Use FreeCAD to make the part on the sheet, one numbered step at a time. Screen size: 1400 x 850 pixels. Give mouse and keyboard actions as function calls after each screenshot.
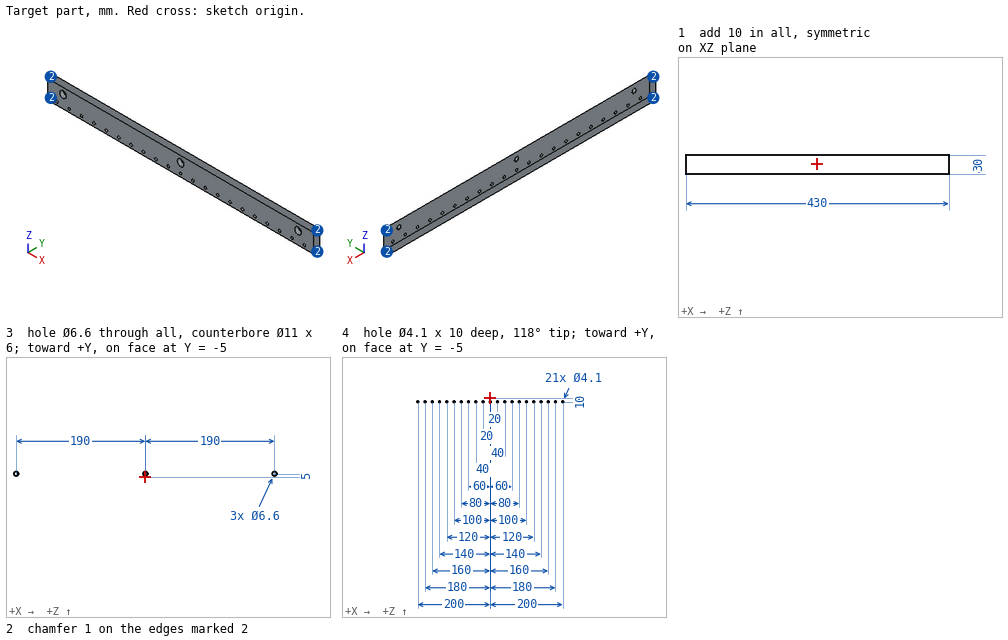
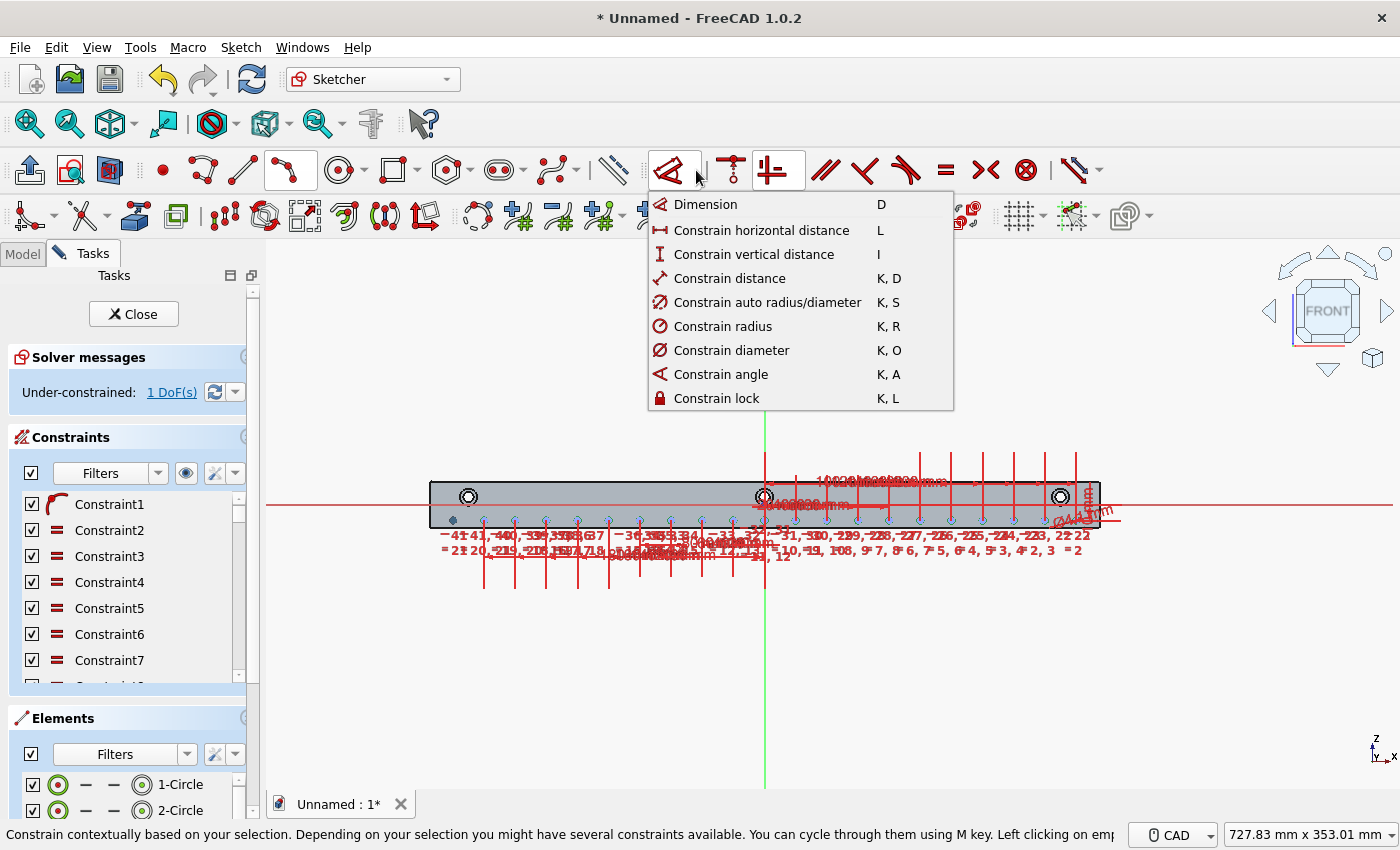
click(801, 230)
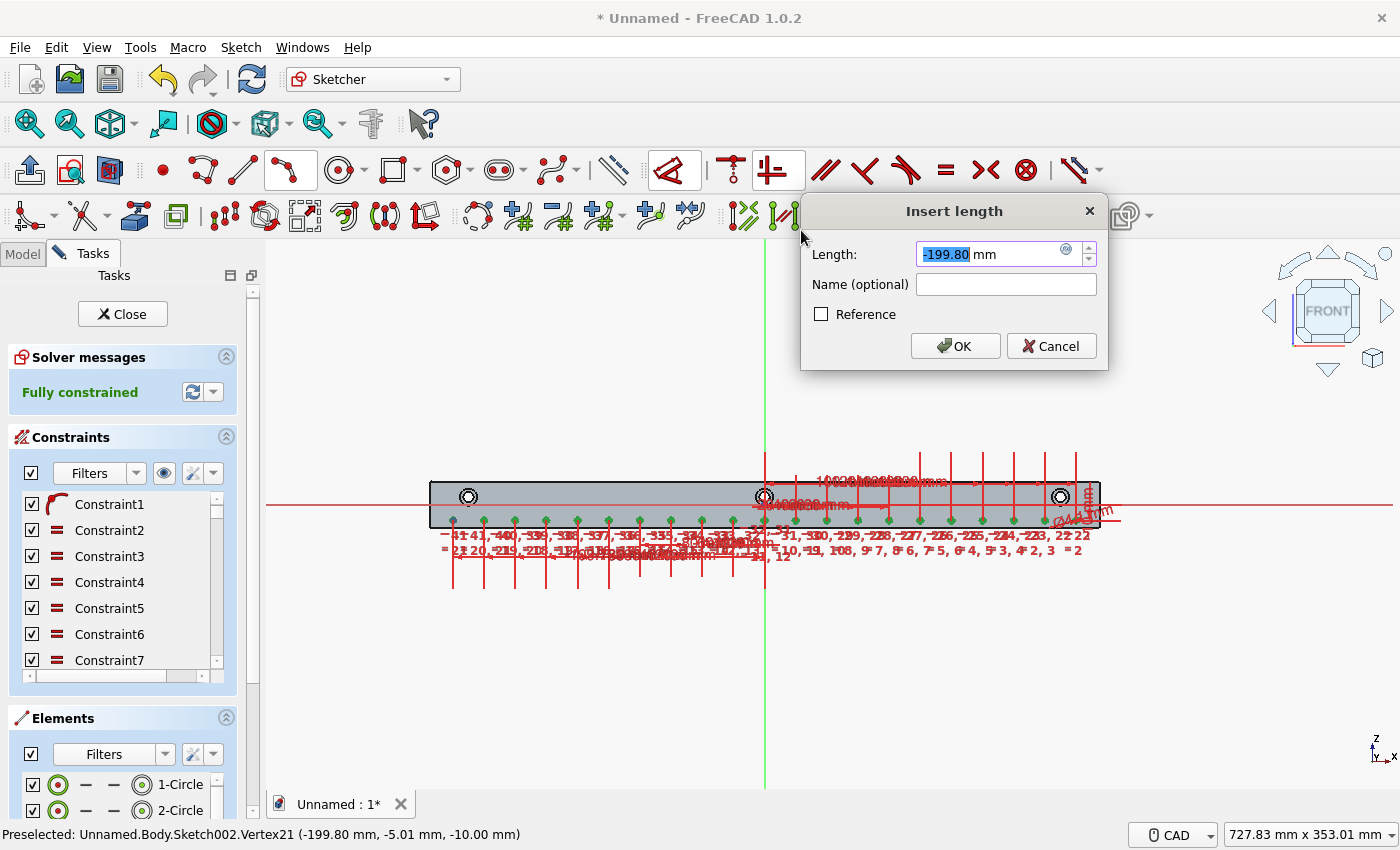
text(-200)
key(Return)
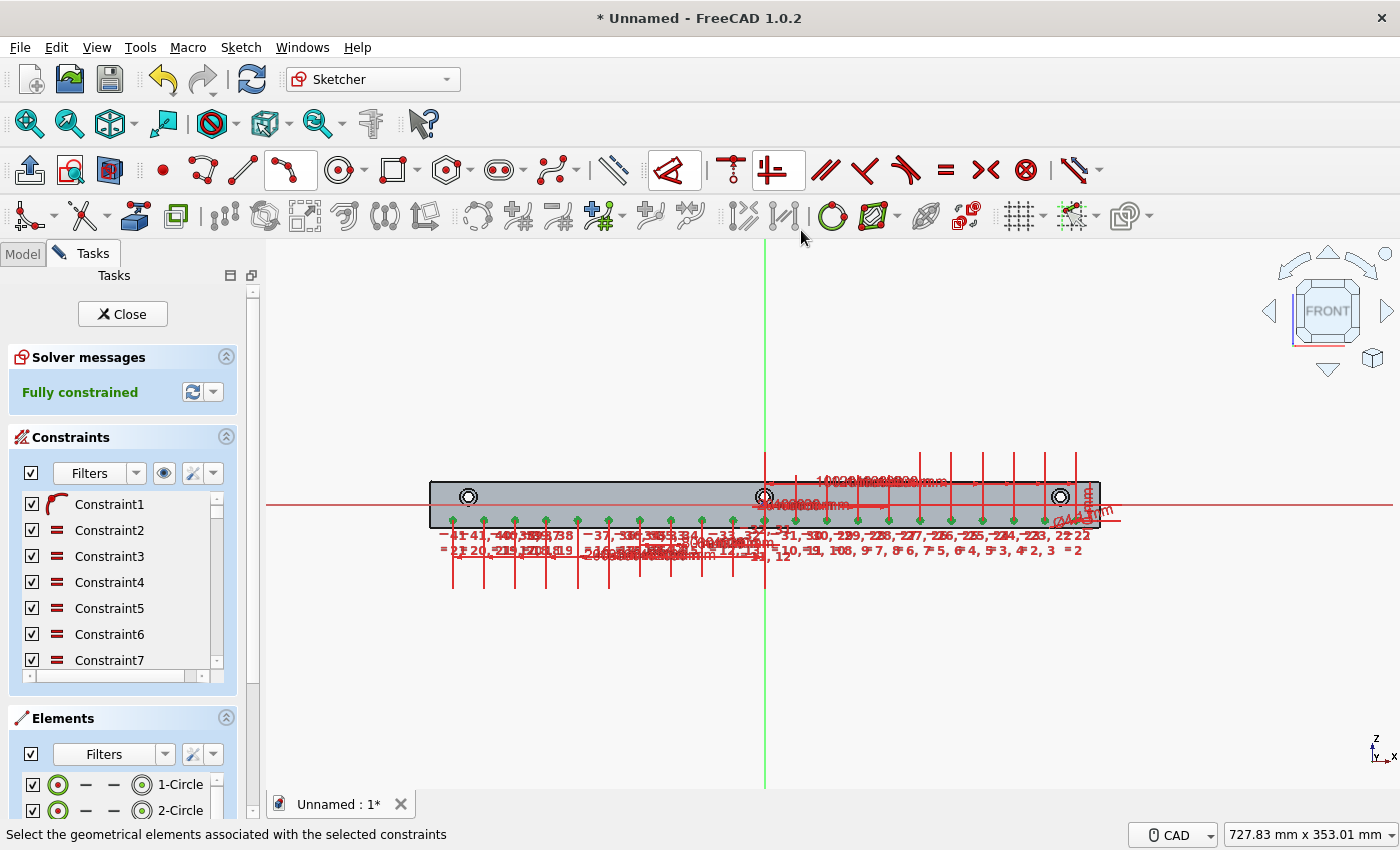
click(123, 314)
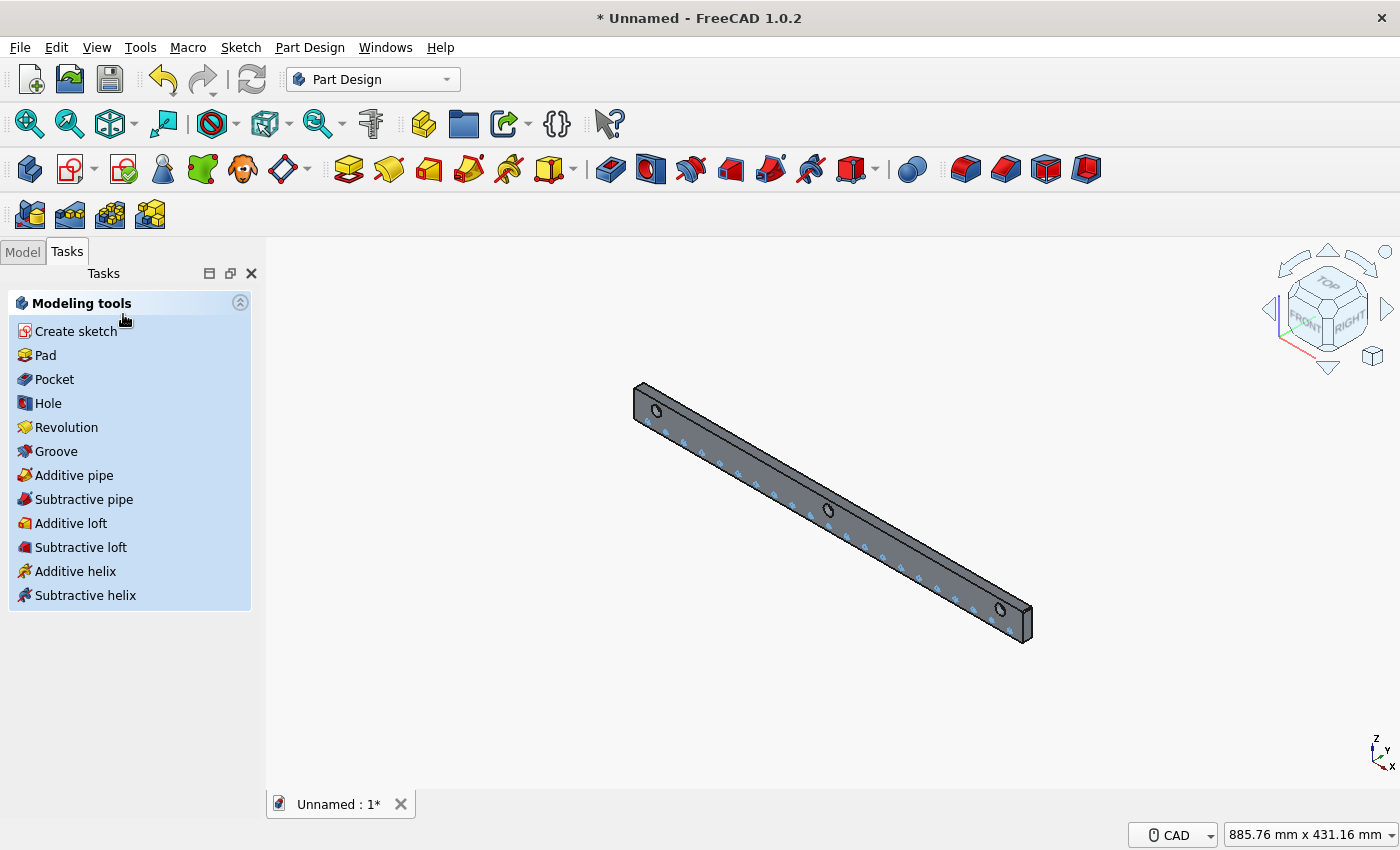
click(652, 170)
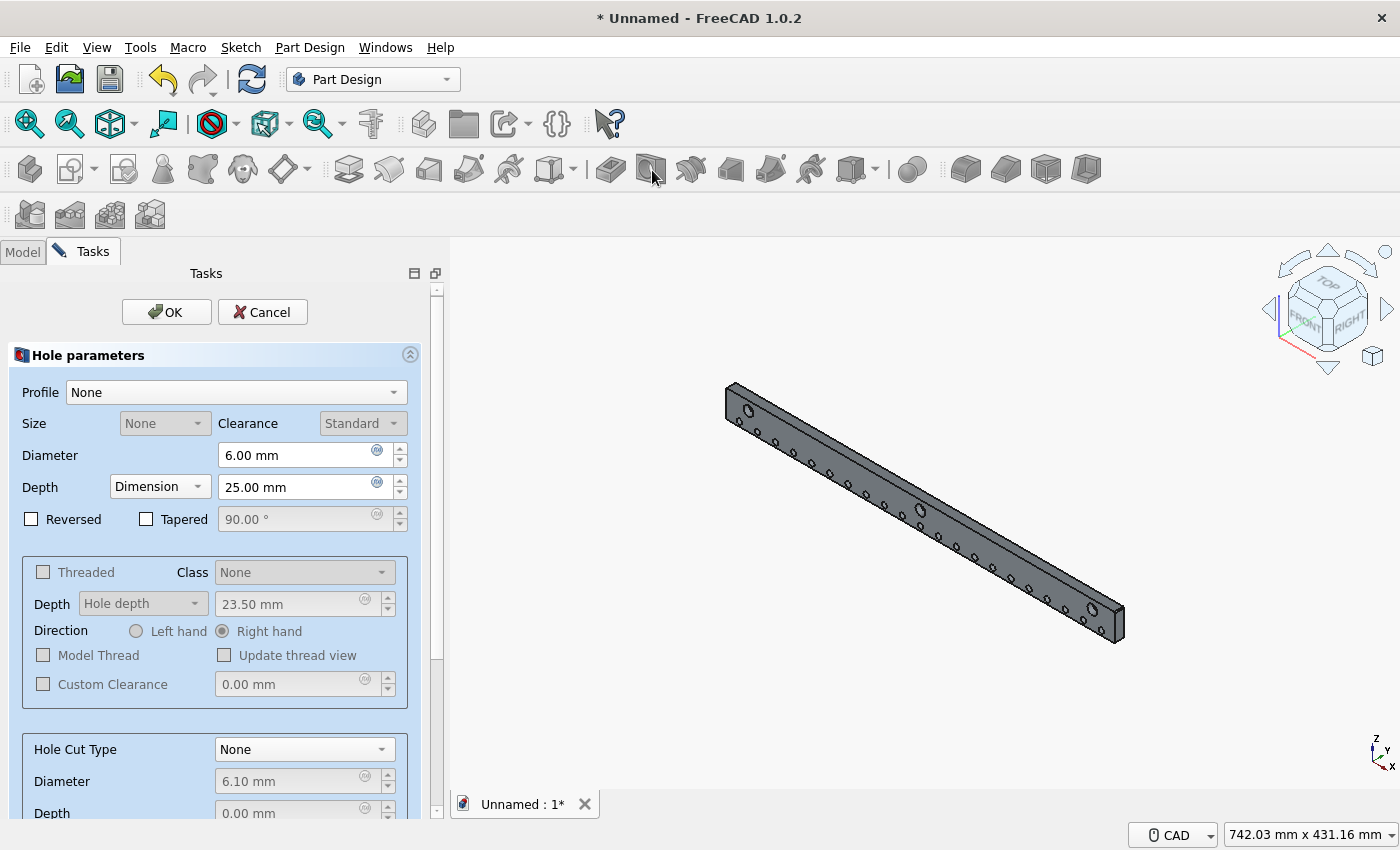
triple_click(305, 455)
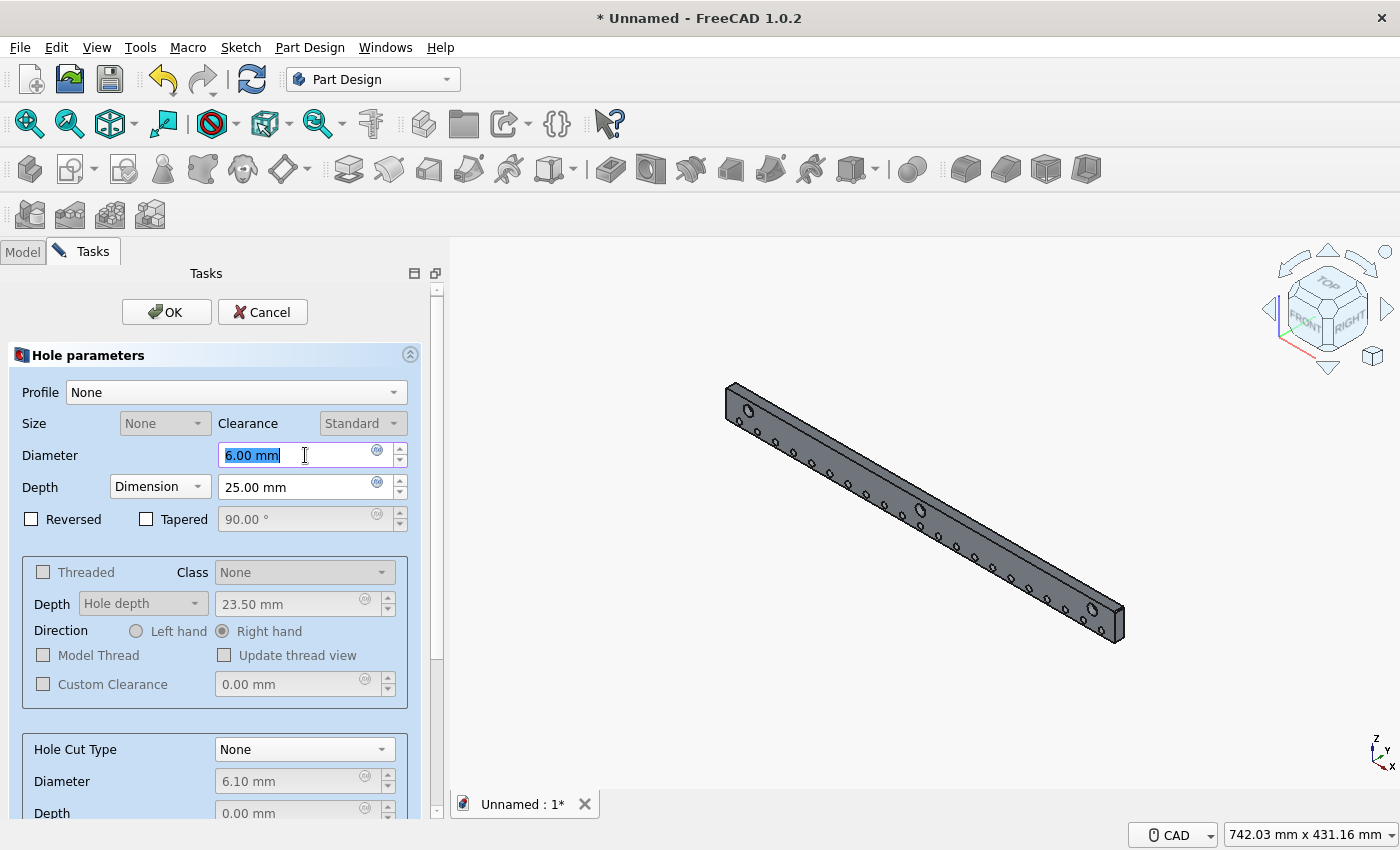
text(4.1)
key(Tab)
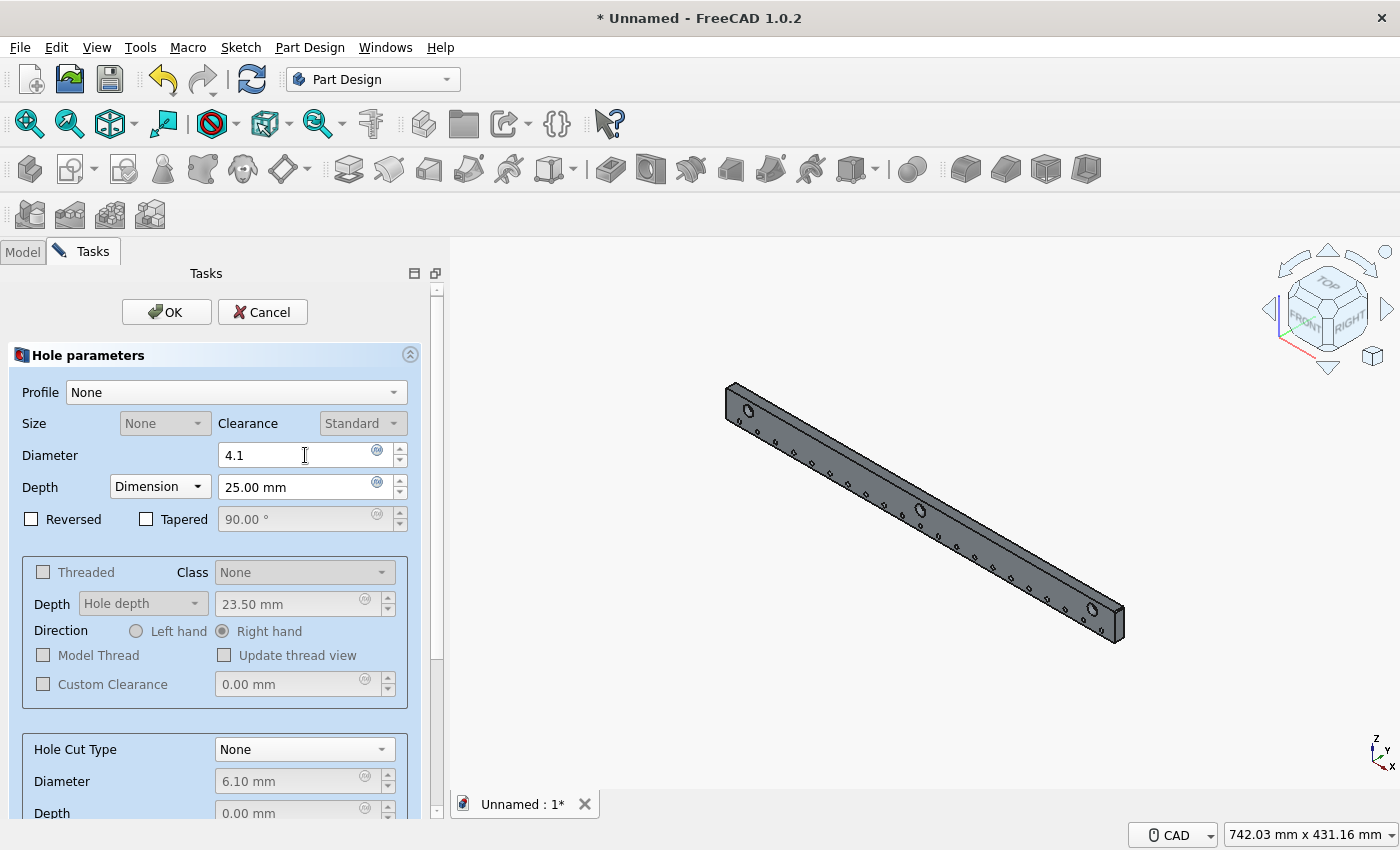
triple_click(305, 487)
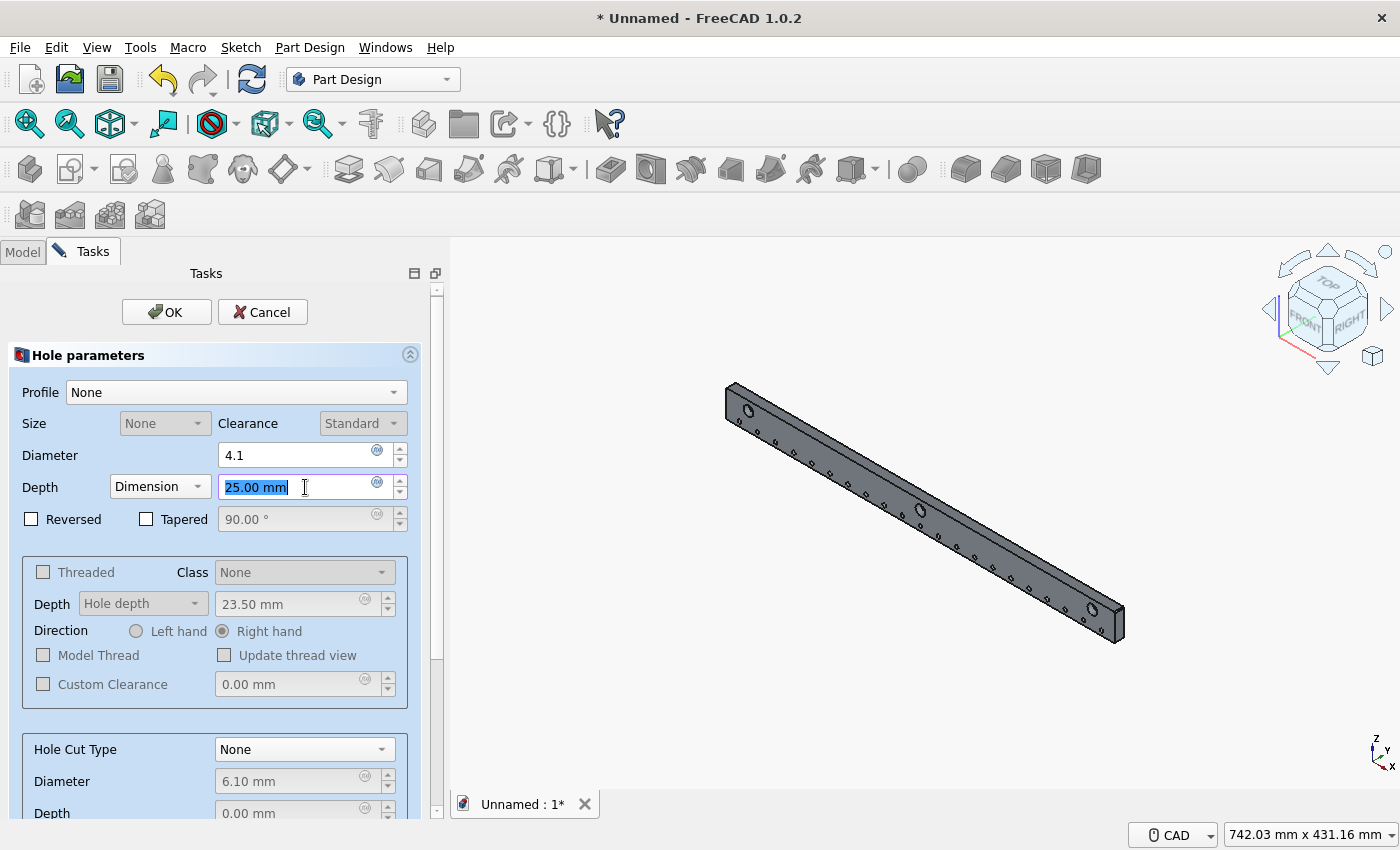
text(10)
key(Tab)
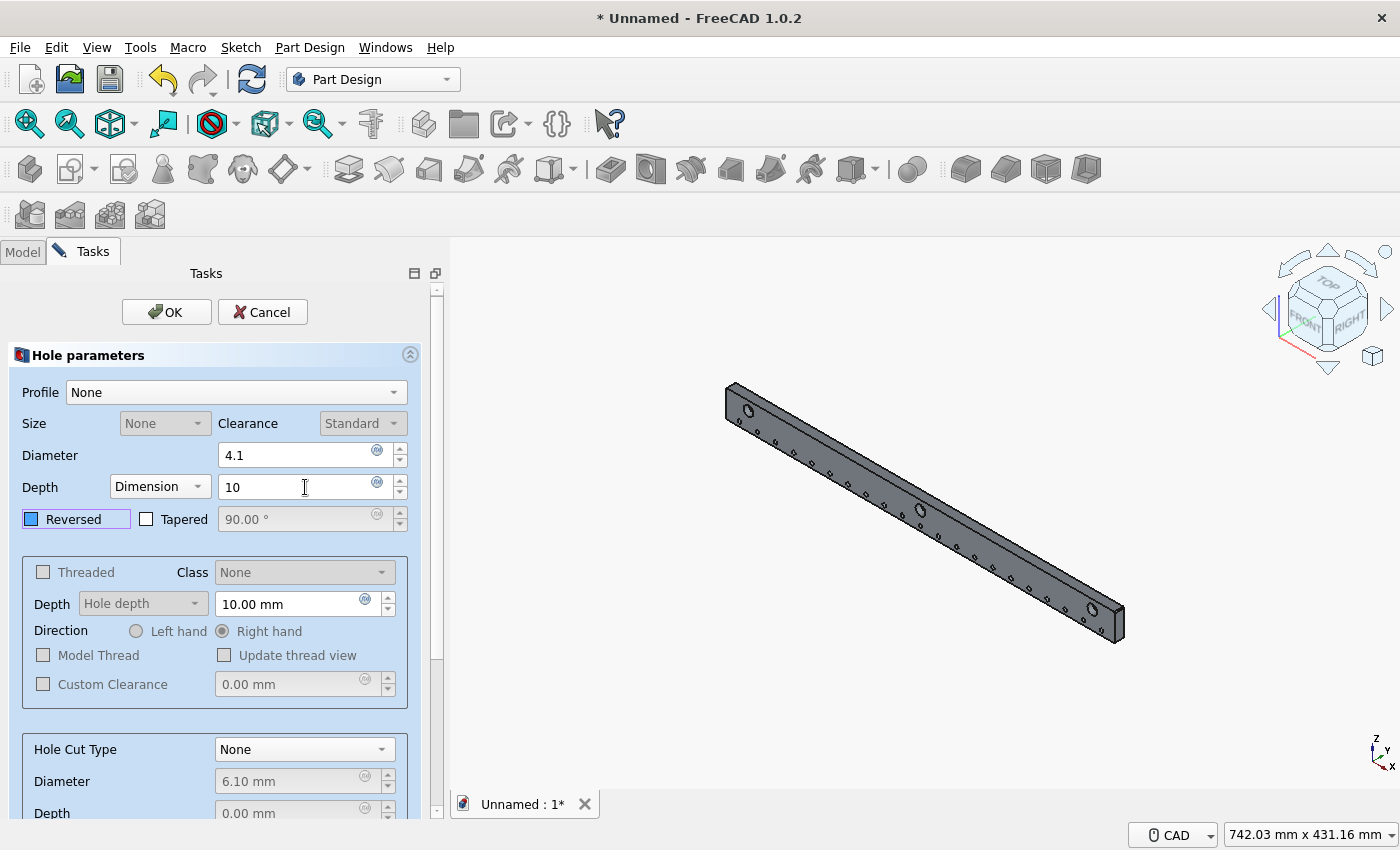
click(167, 312)